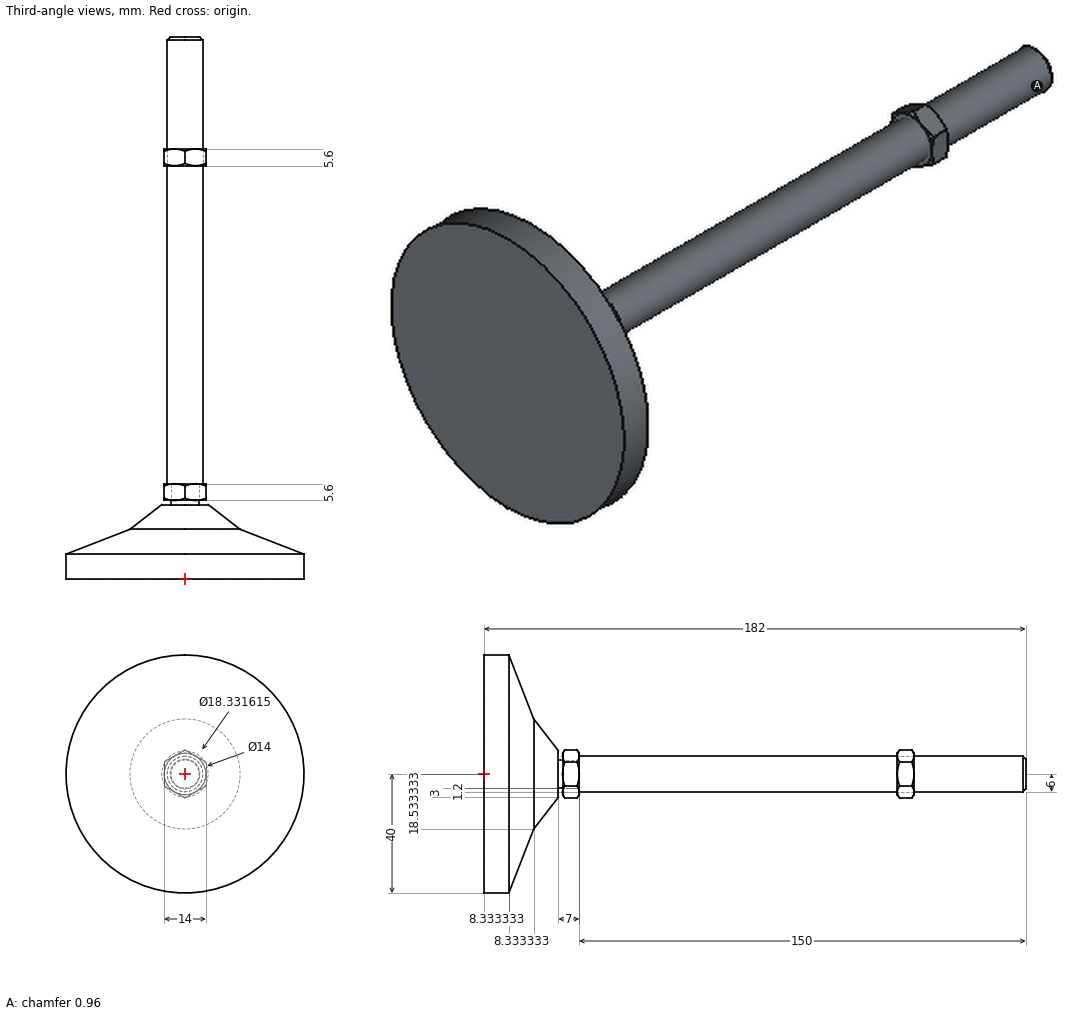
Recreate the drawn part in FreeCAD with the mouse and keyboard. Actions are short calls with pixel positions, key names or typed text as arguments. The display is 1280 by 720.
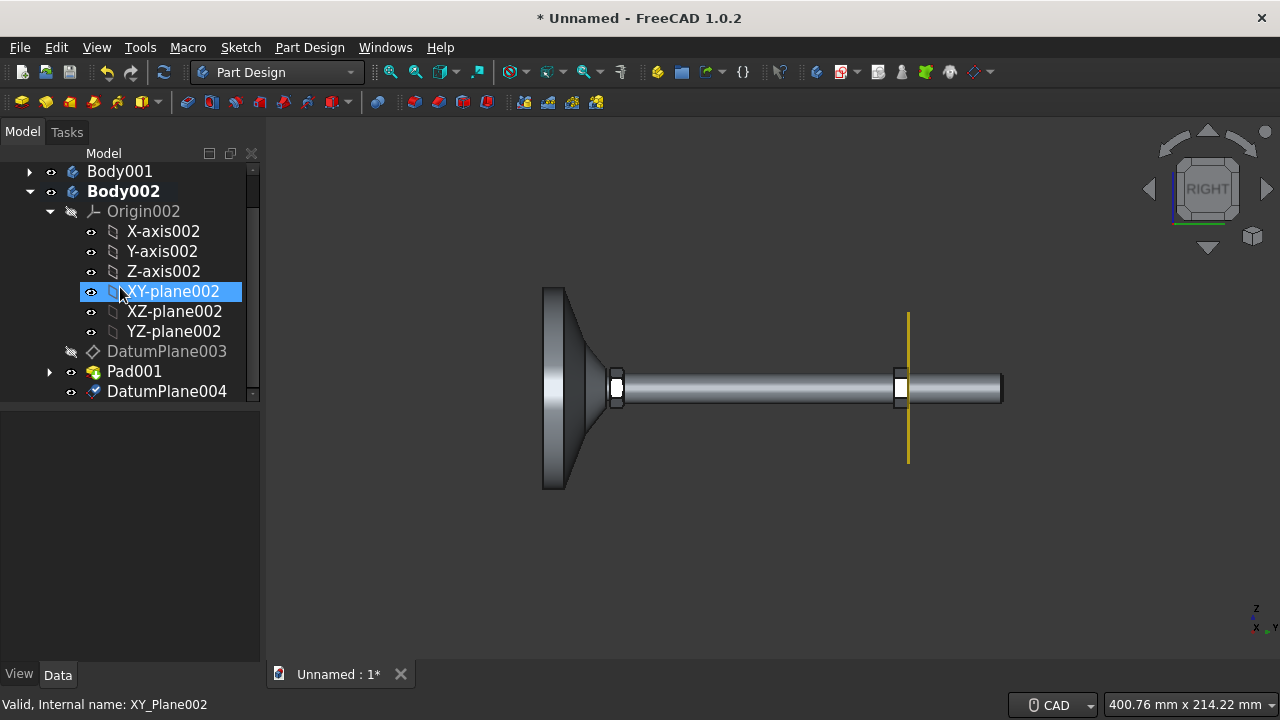
click(116, 392)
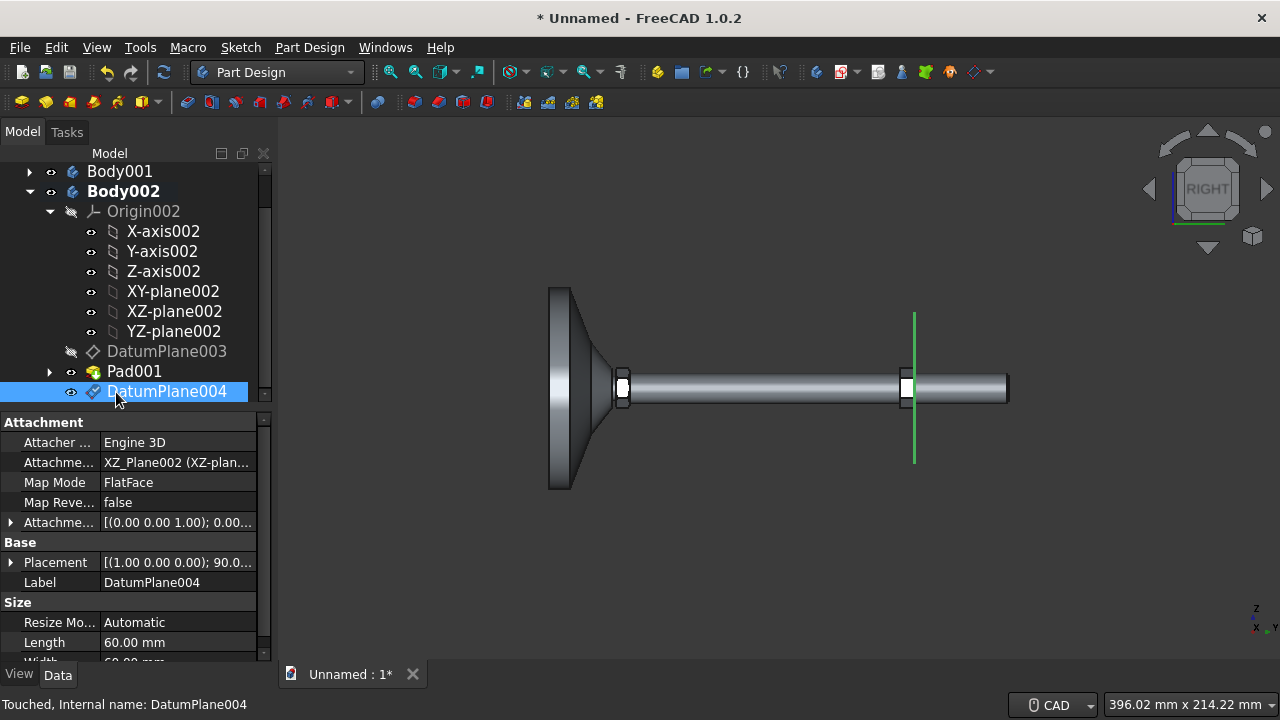
click(842, 72)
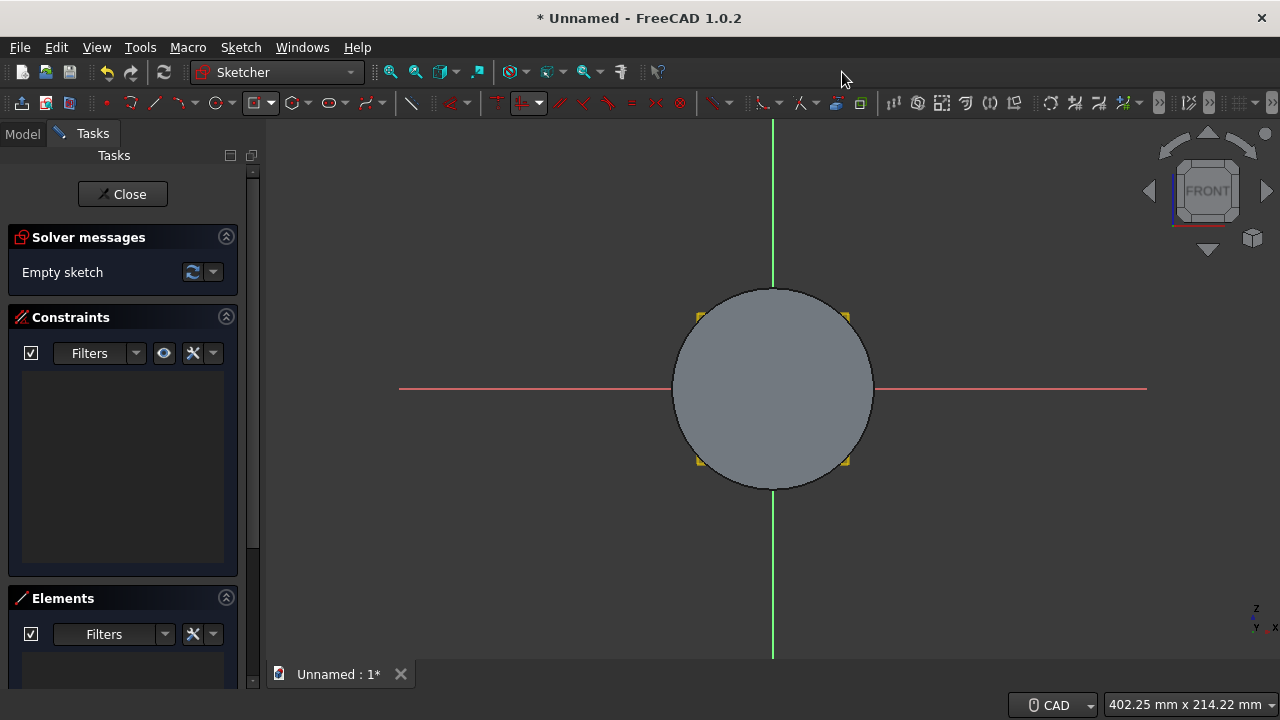
key(q)
key(s)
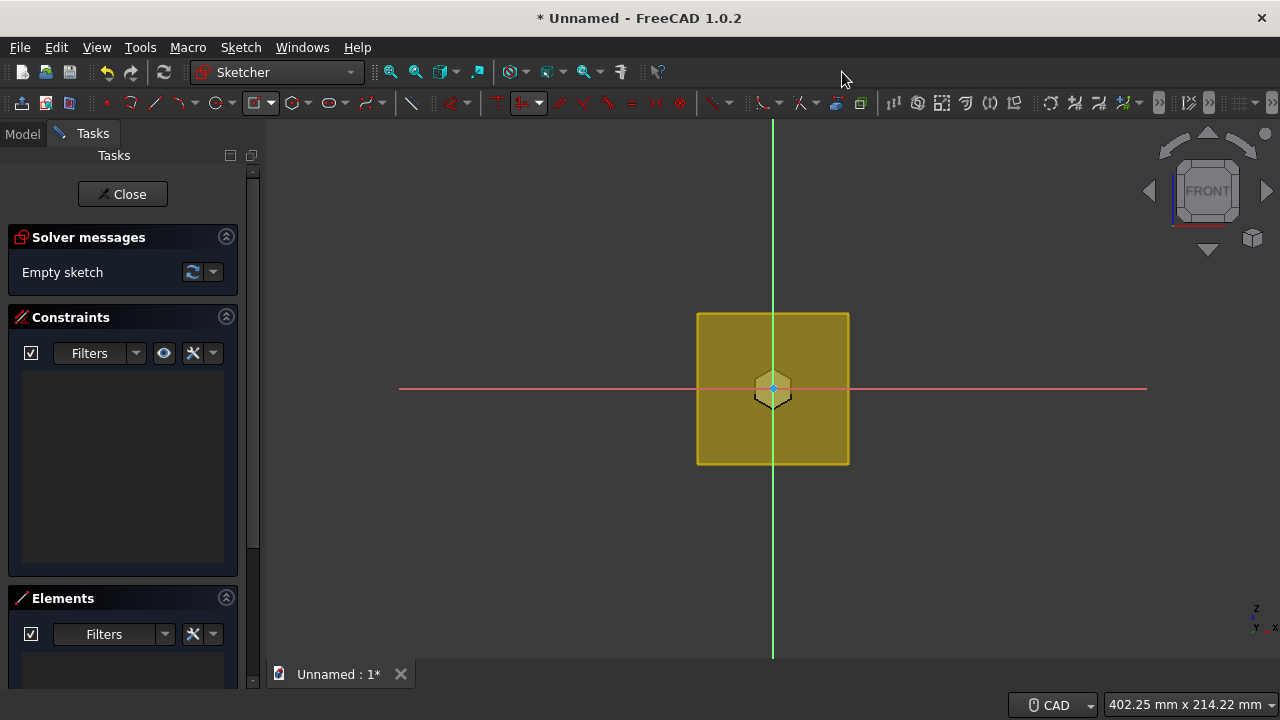
scroll(784, 389, up, 10)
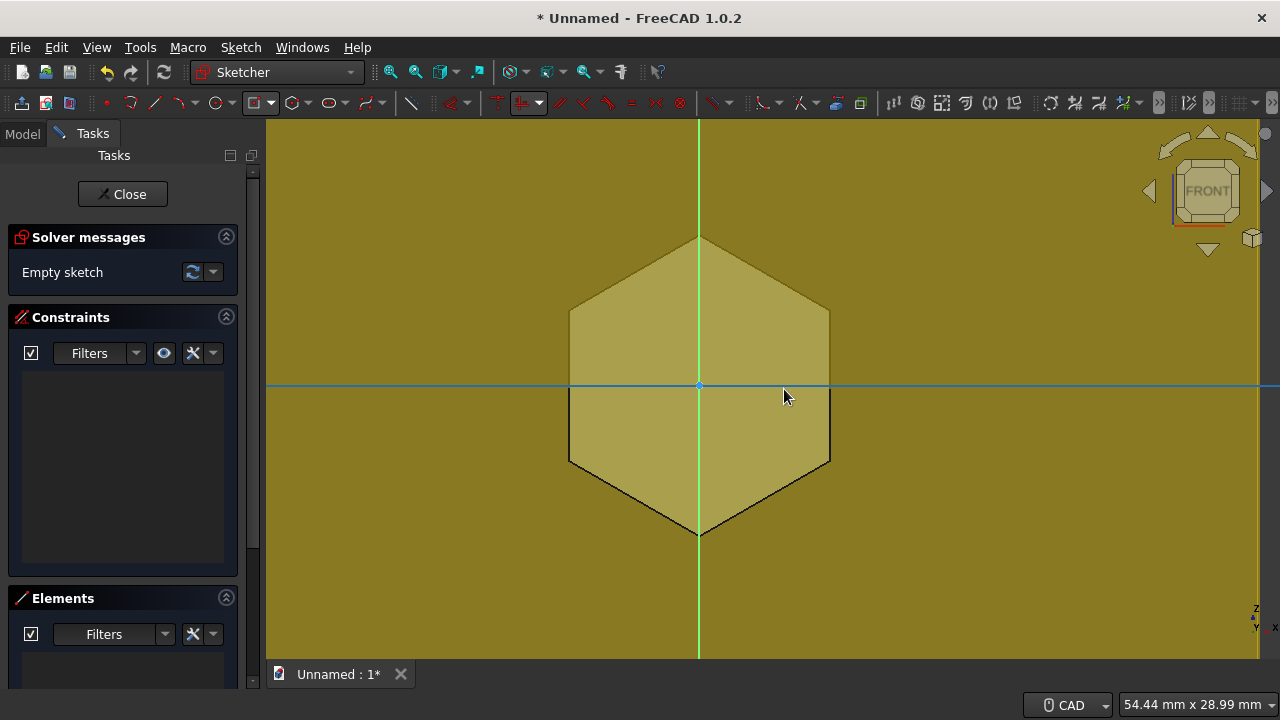
click(216, 104)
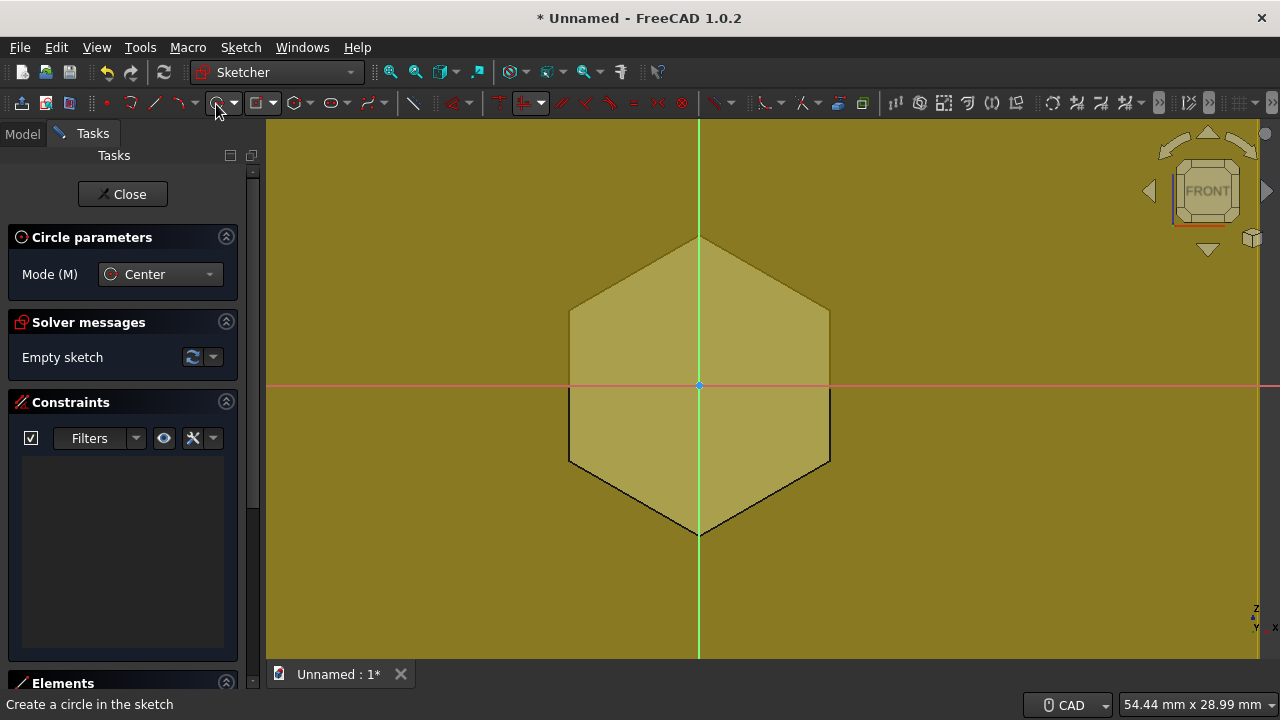
click(699, 386)
click(820, 265)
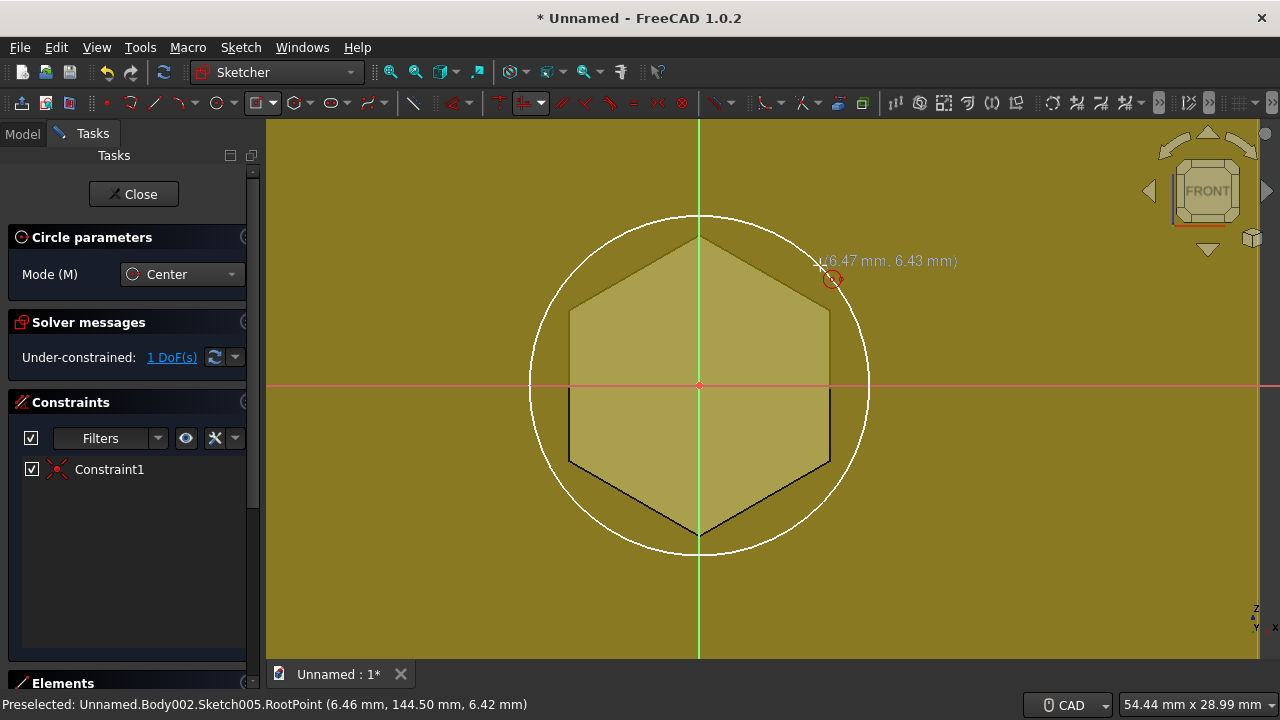
click(699, 386)
click(792, 294)
key(Escape)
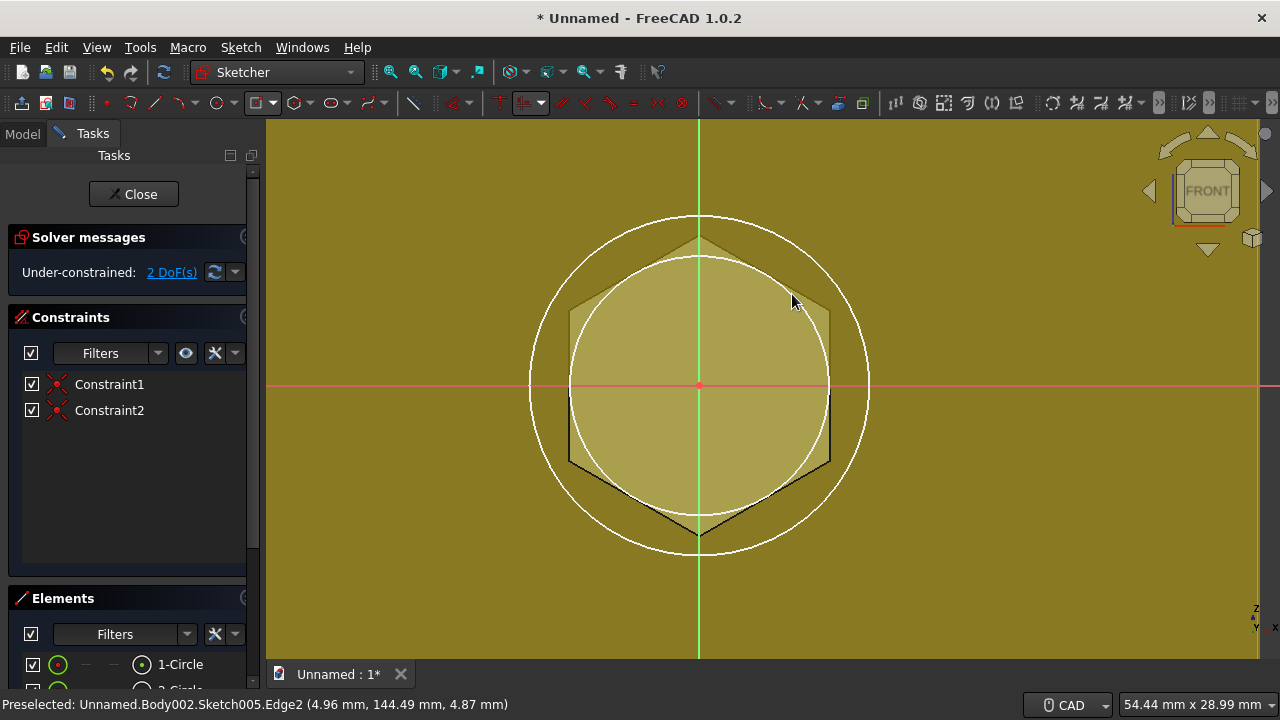
key(d)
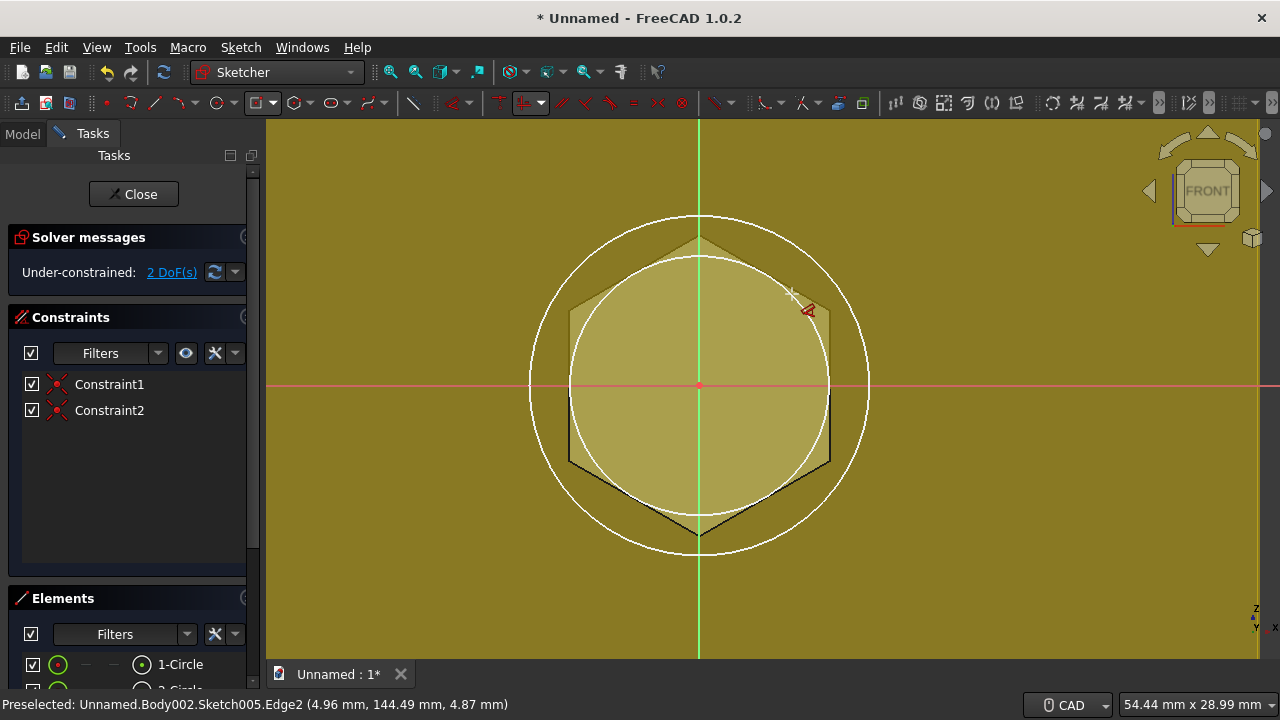
click(819, 265)
click(842, 242)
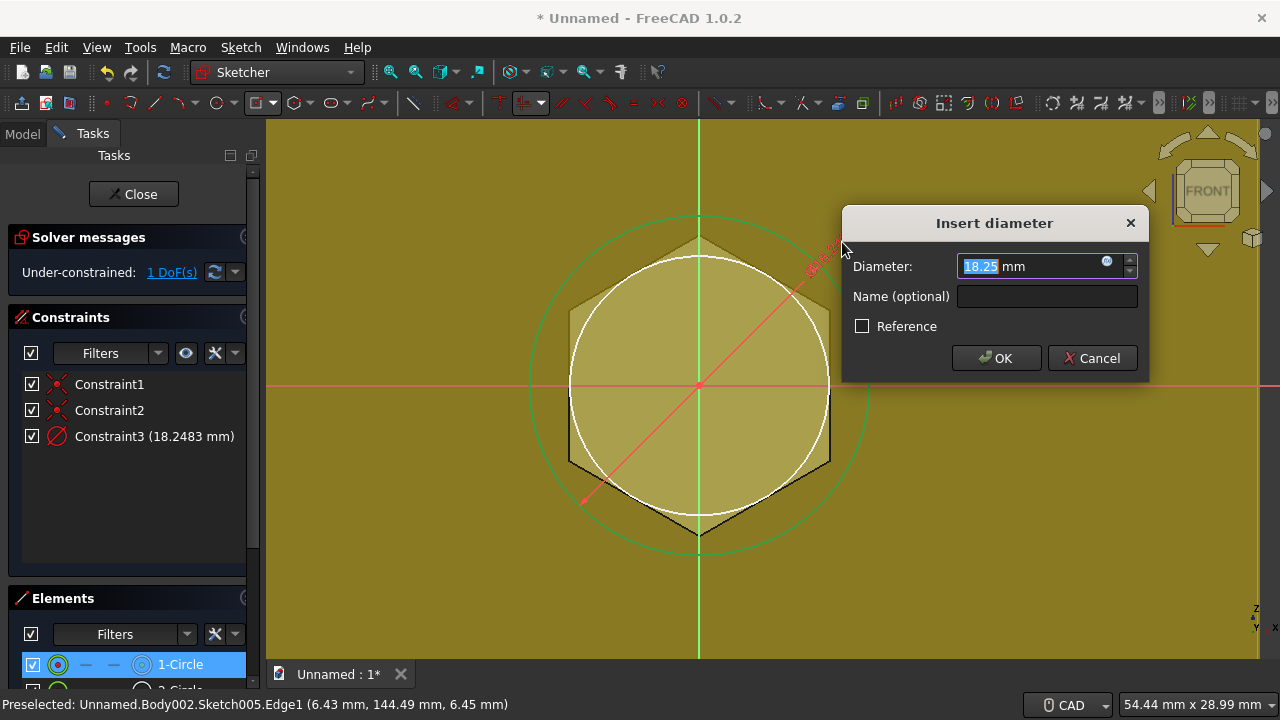
text(18.331615)
key(Return)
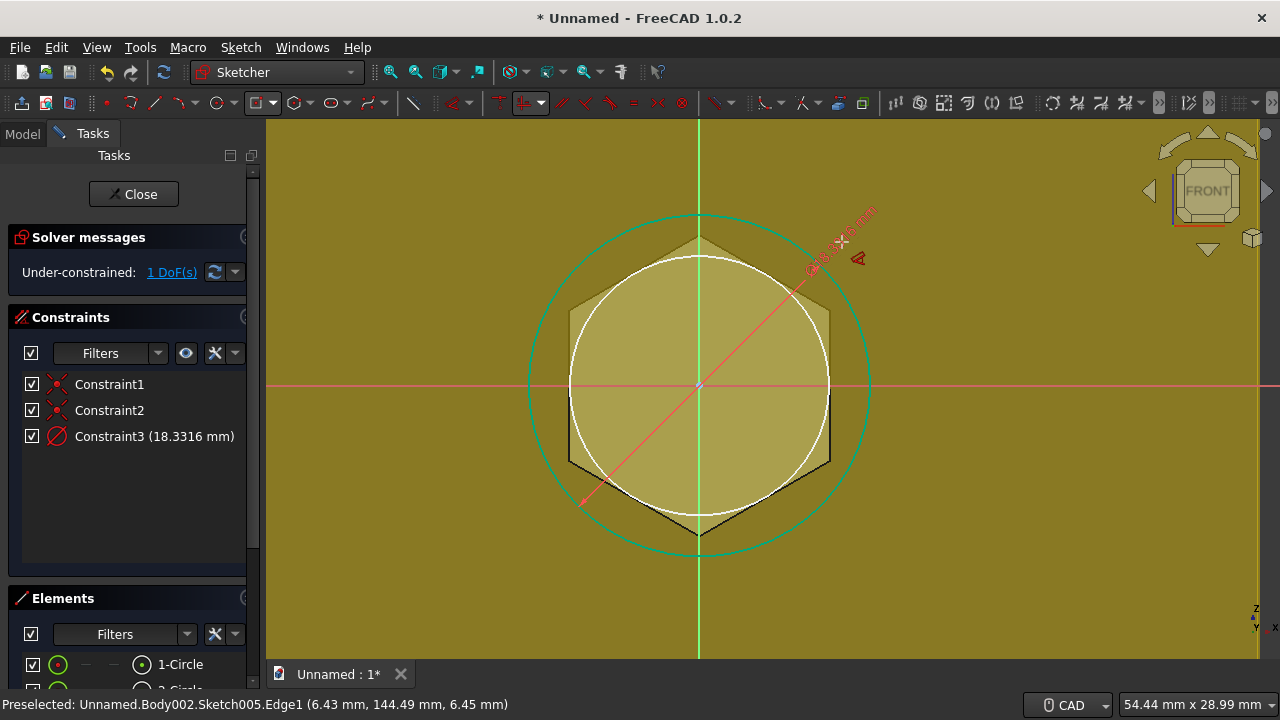
click(791, 294)
click(877, 334)